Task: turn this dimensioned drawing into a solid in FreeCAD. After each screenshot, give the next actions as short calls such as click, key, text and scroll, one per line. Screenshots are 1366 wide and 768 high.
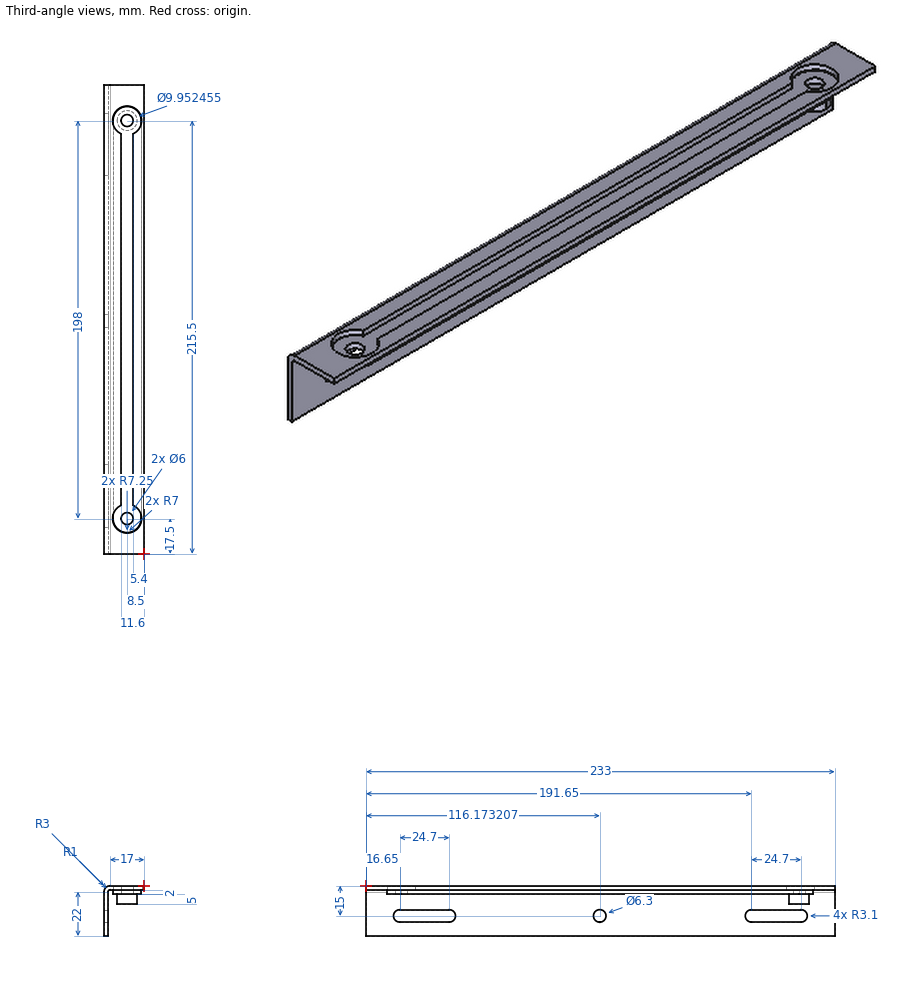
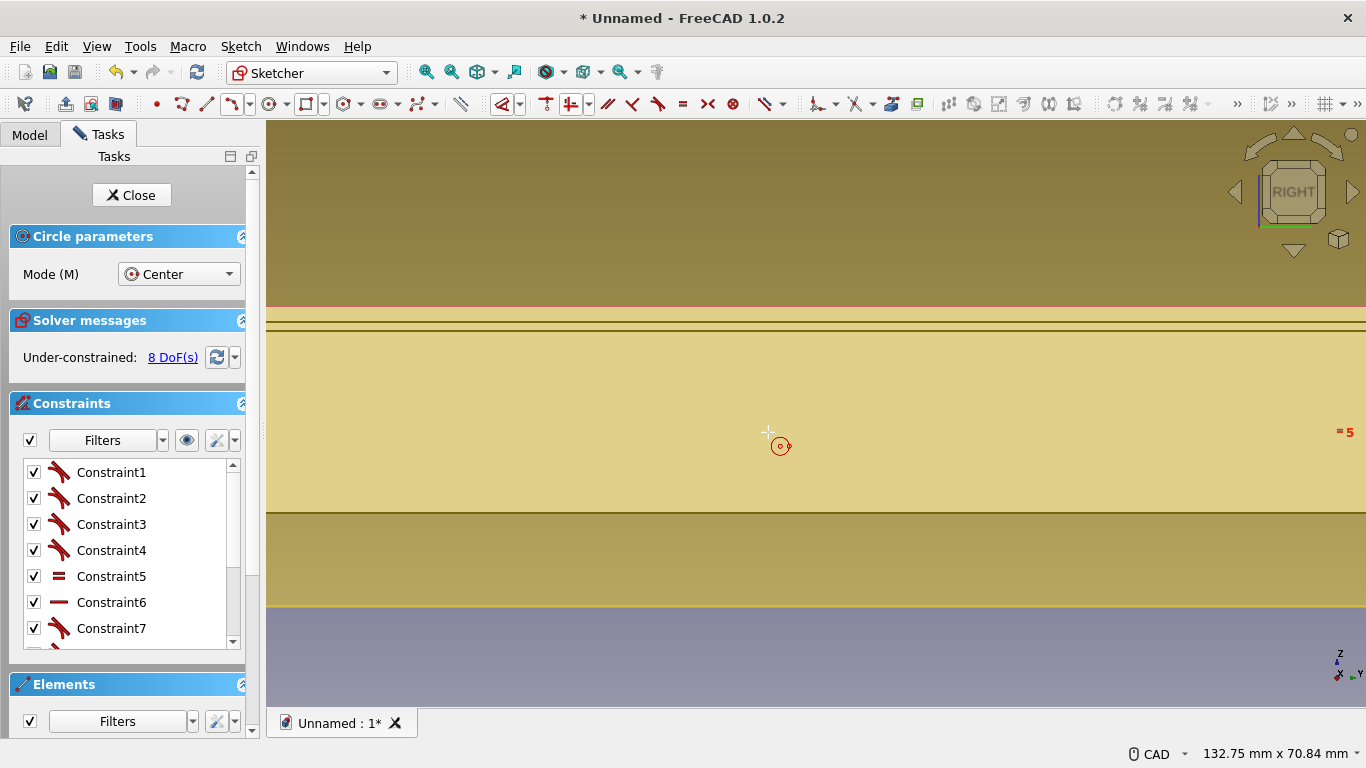
click(766, 430)
click(784, 412)
key(Escape)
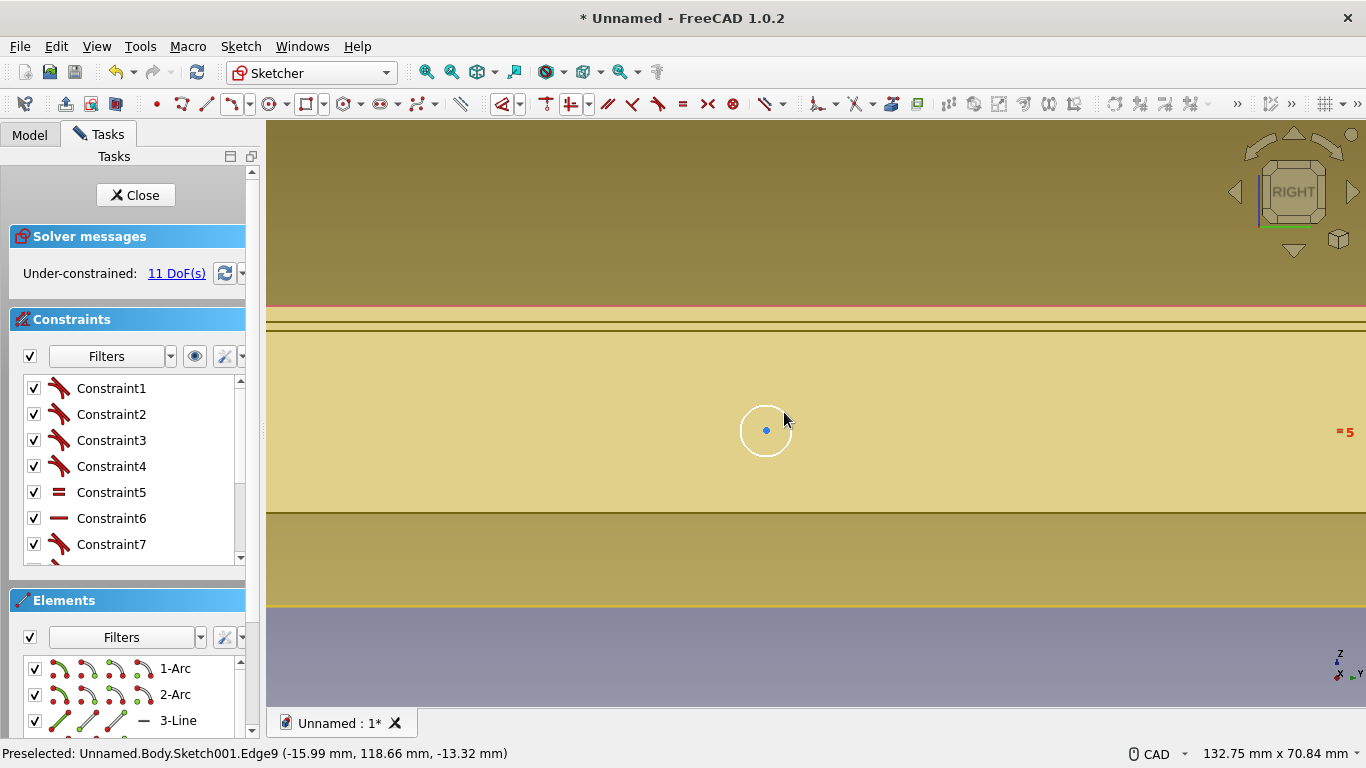
scroll(768, 432, down, 5)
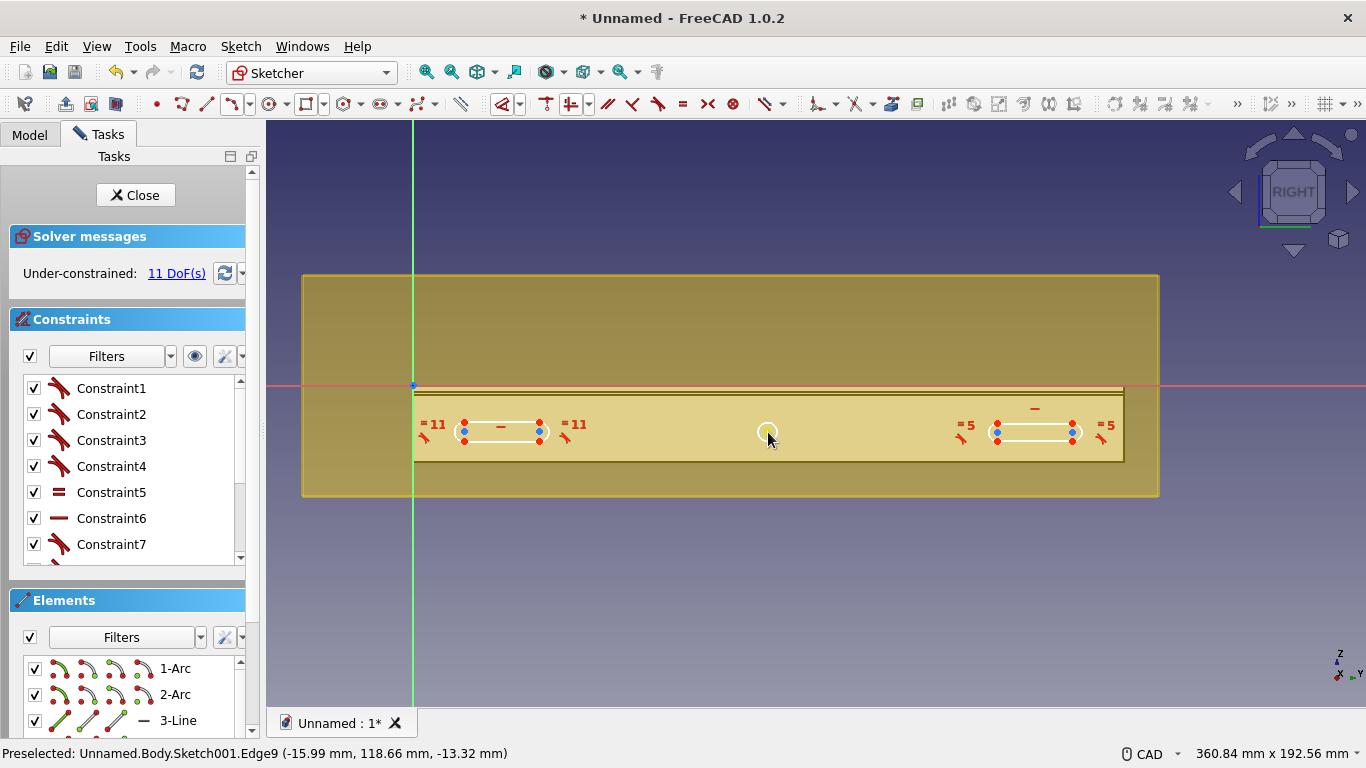
scroll(991, 427, up, 3)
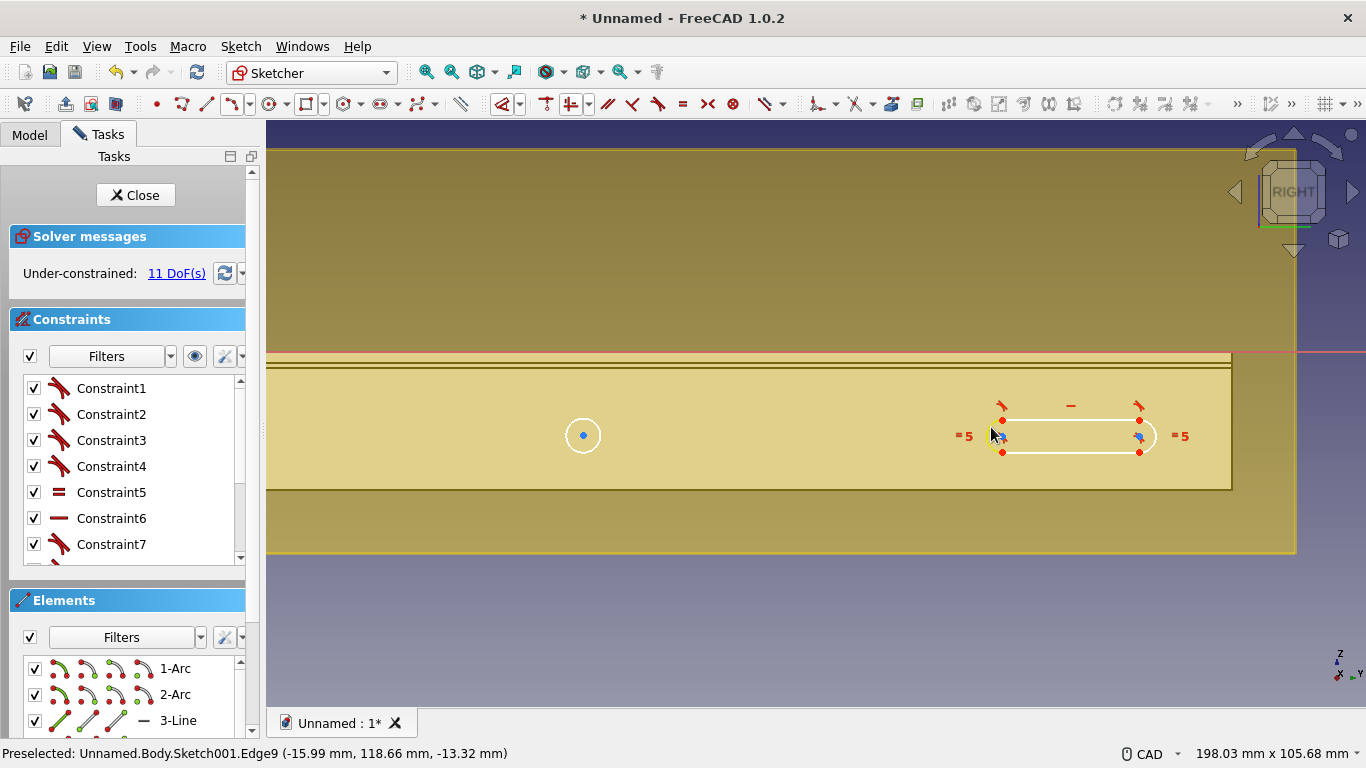
click(990, 427)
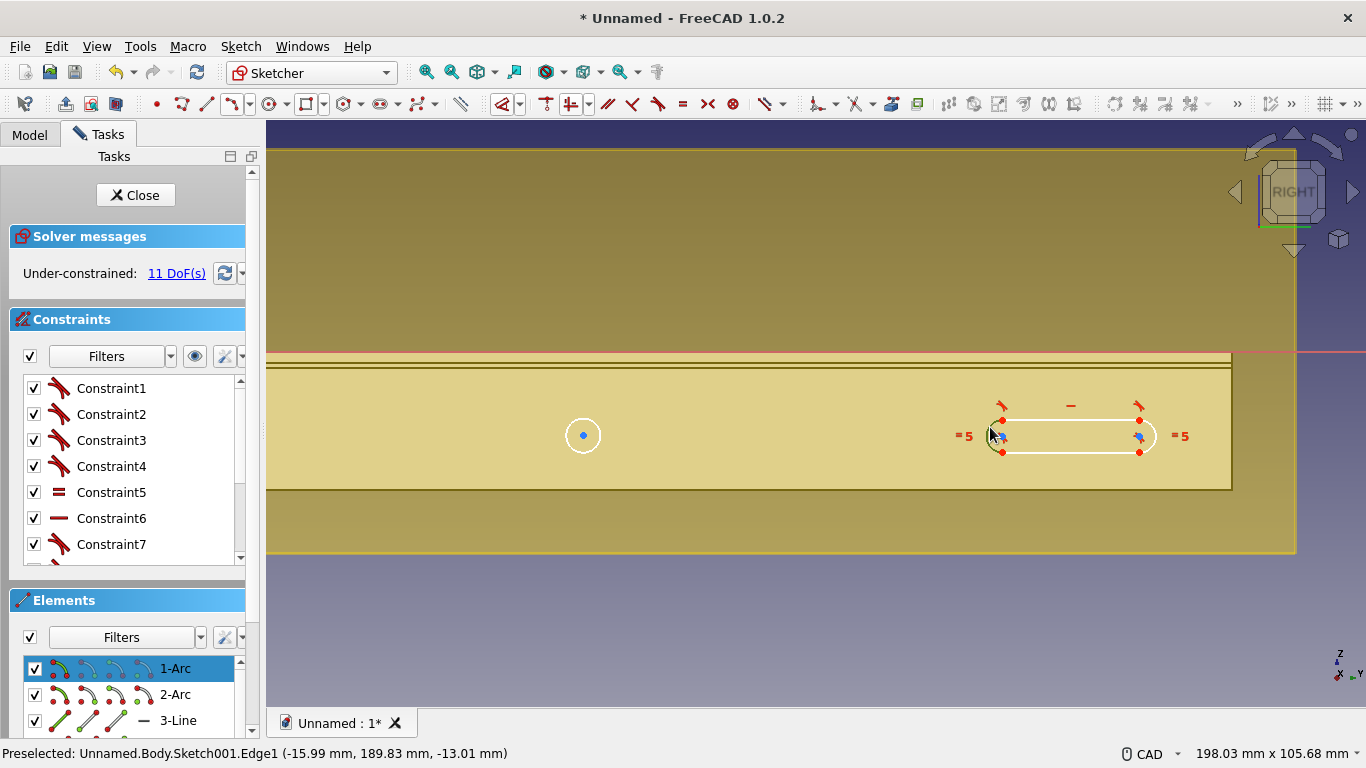
scroll(991, 427, down, 3)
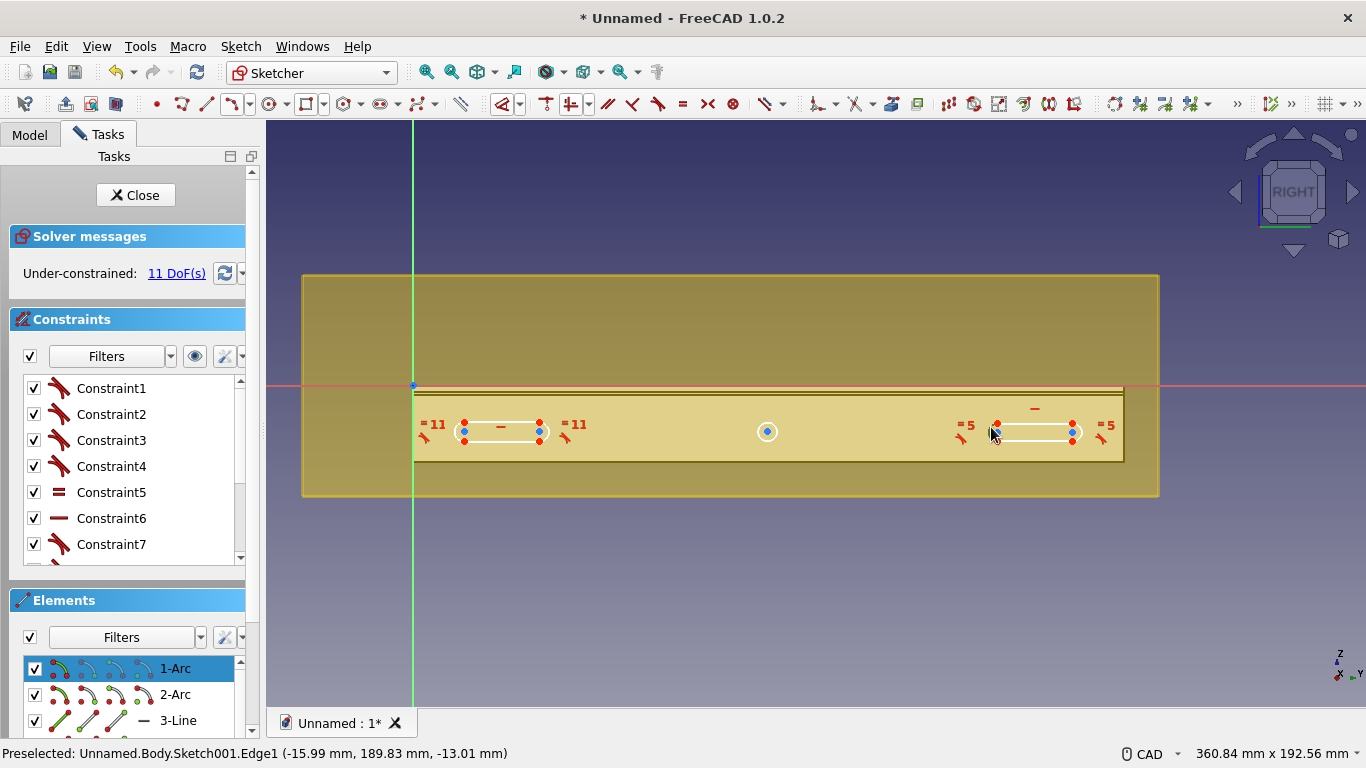
scroll(456, 426, up, 3)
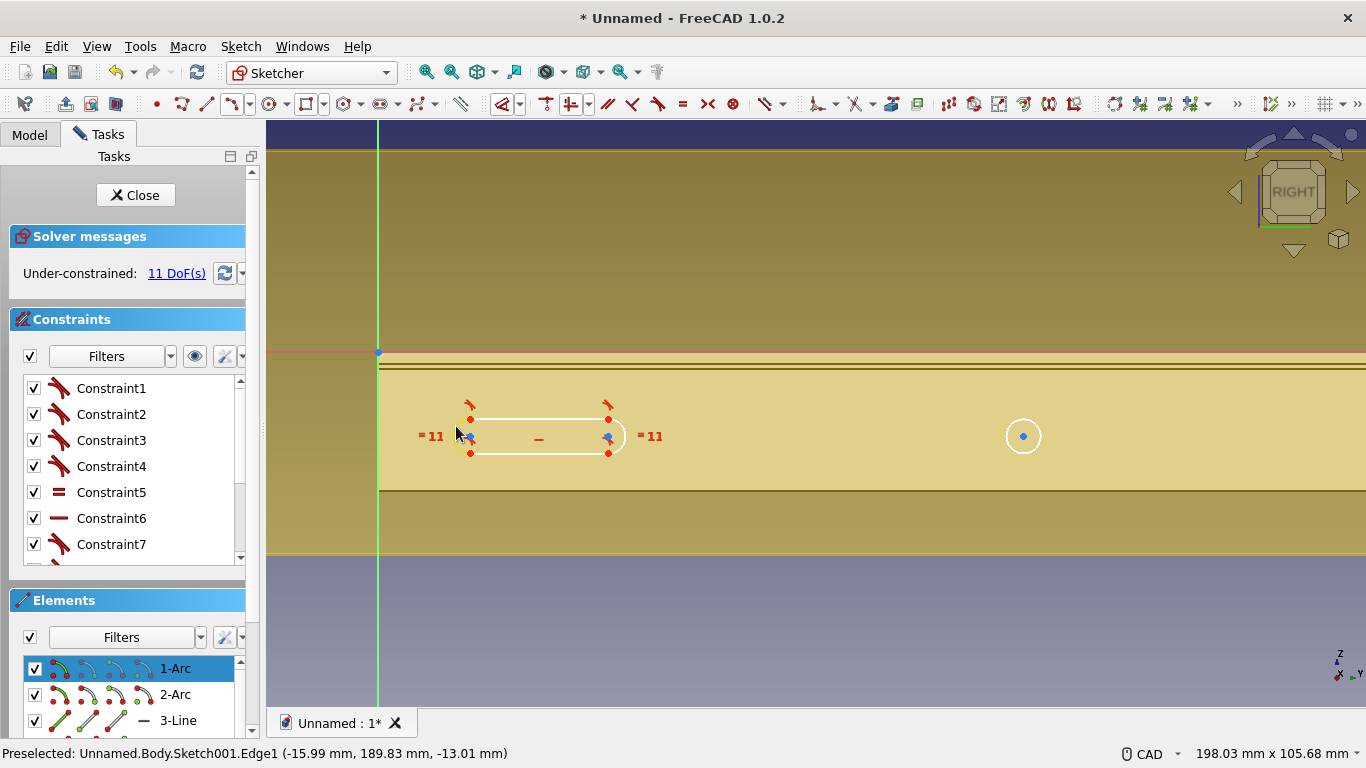
click(457, 426)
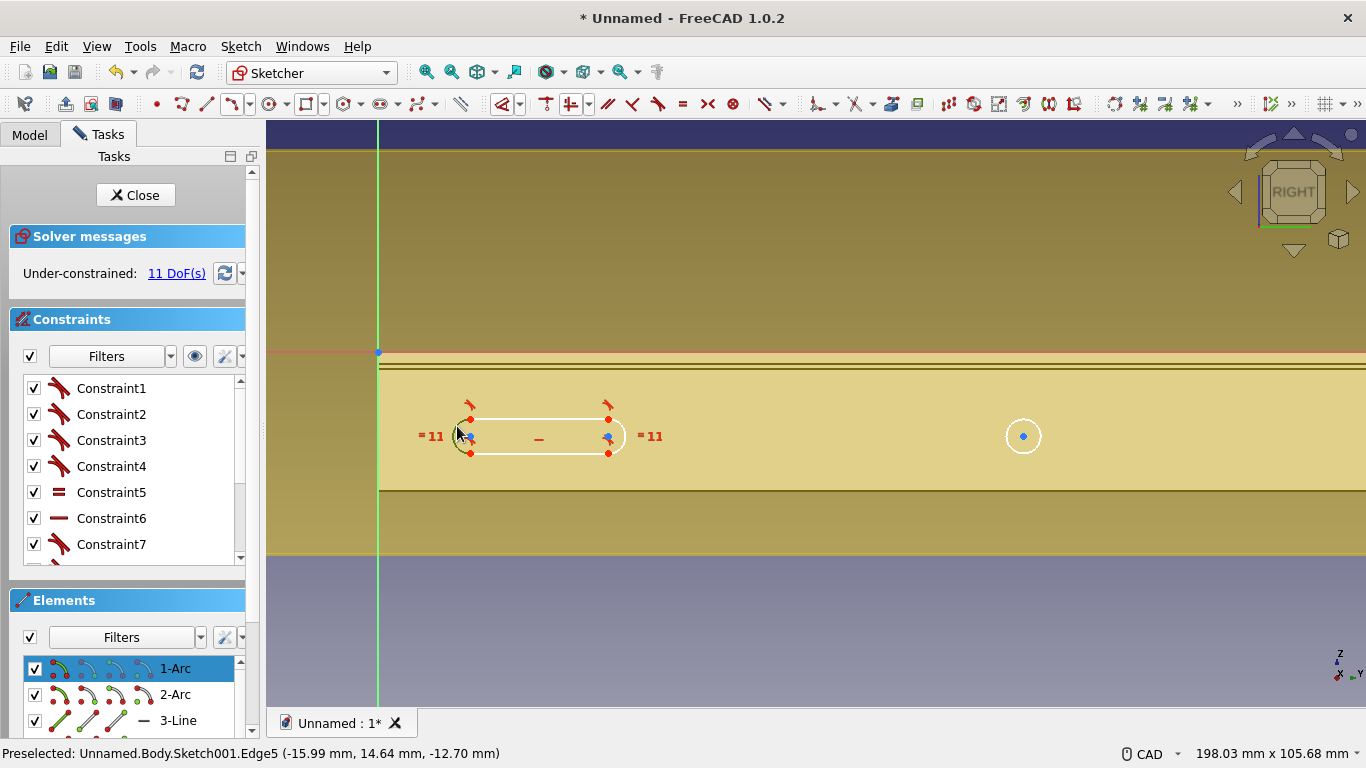
click(683, 104)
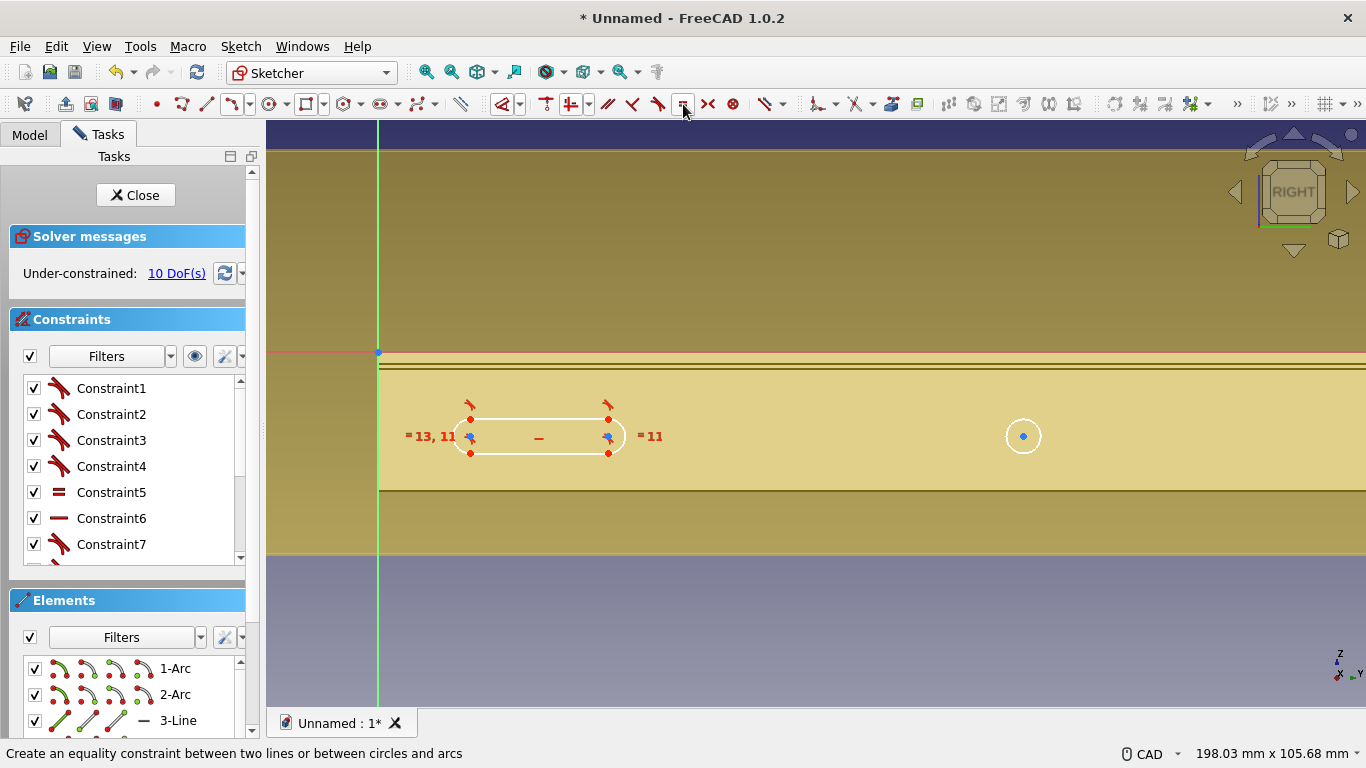
scroll(455, 426, down, 3)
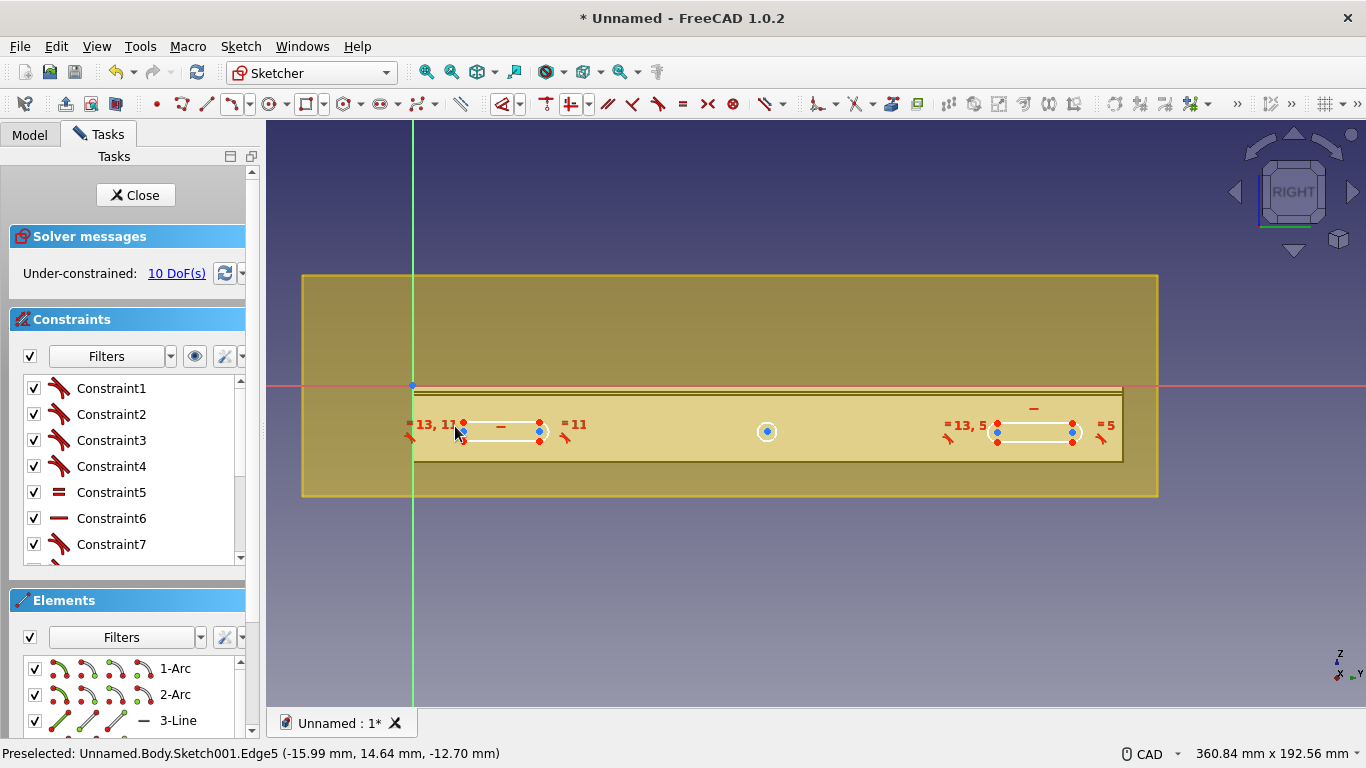
scroll(990, 427, up, 8)